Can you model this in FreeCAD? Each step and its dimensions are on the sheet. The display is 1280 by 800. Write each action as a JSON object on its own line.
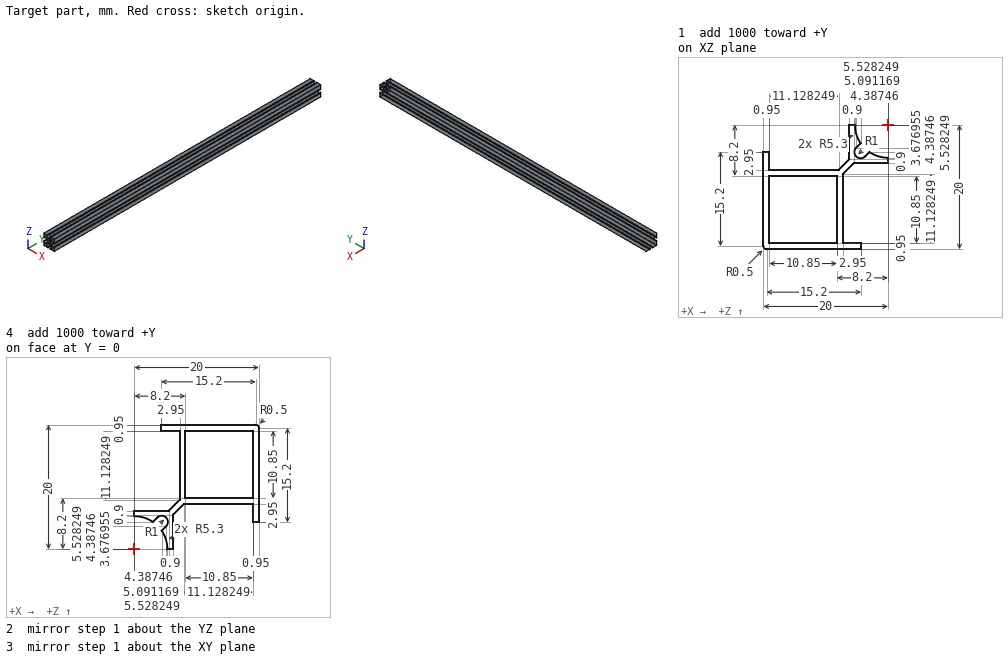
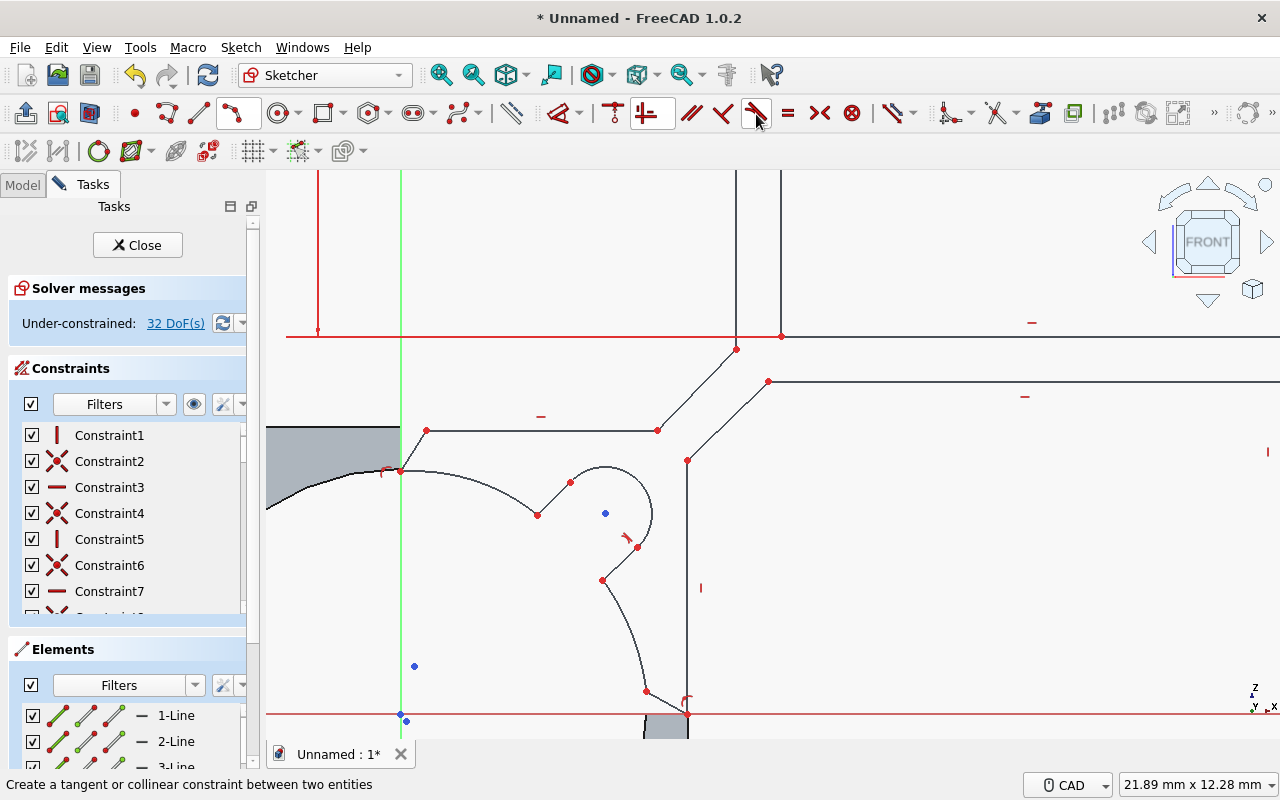
{"action": "left_click", "coordinate": [561, 492]}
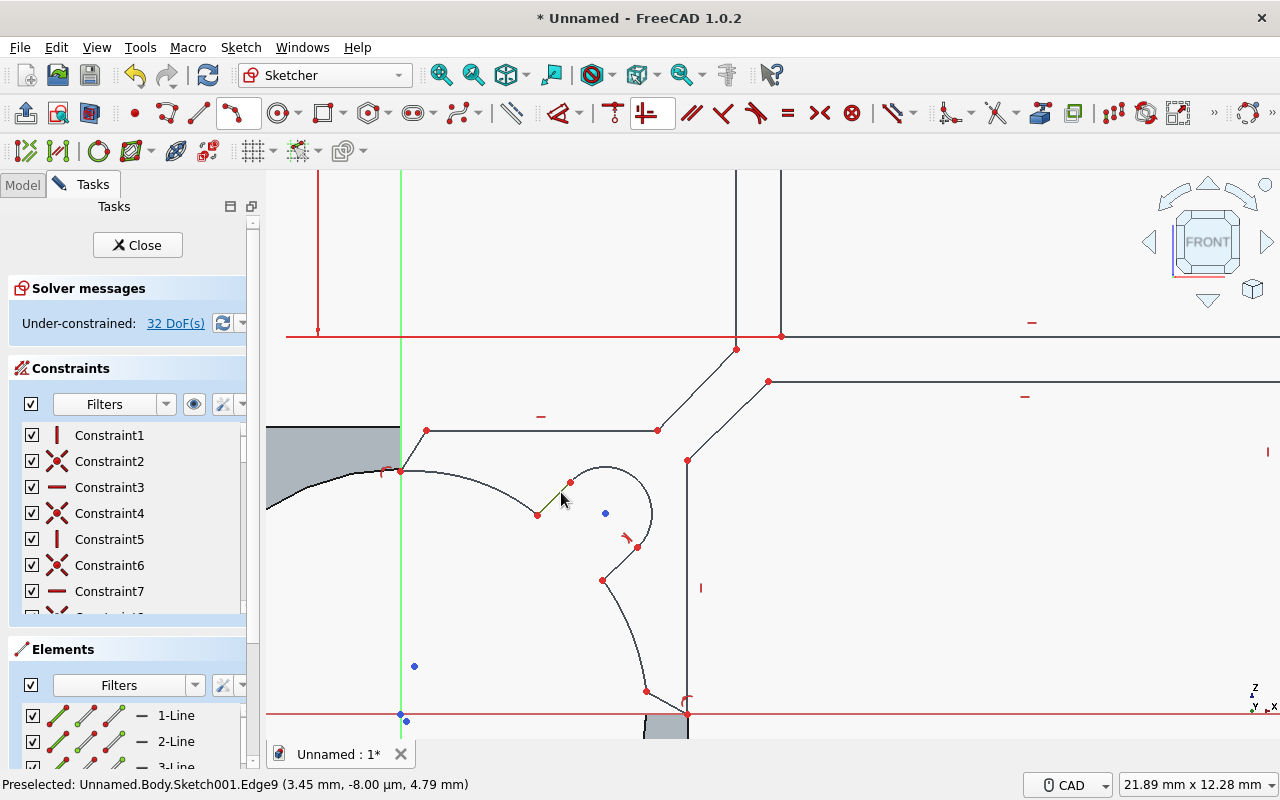
{"action": "left_click", "coordinate": [651, 507]}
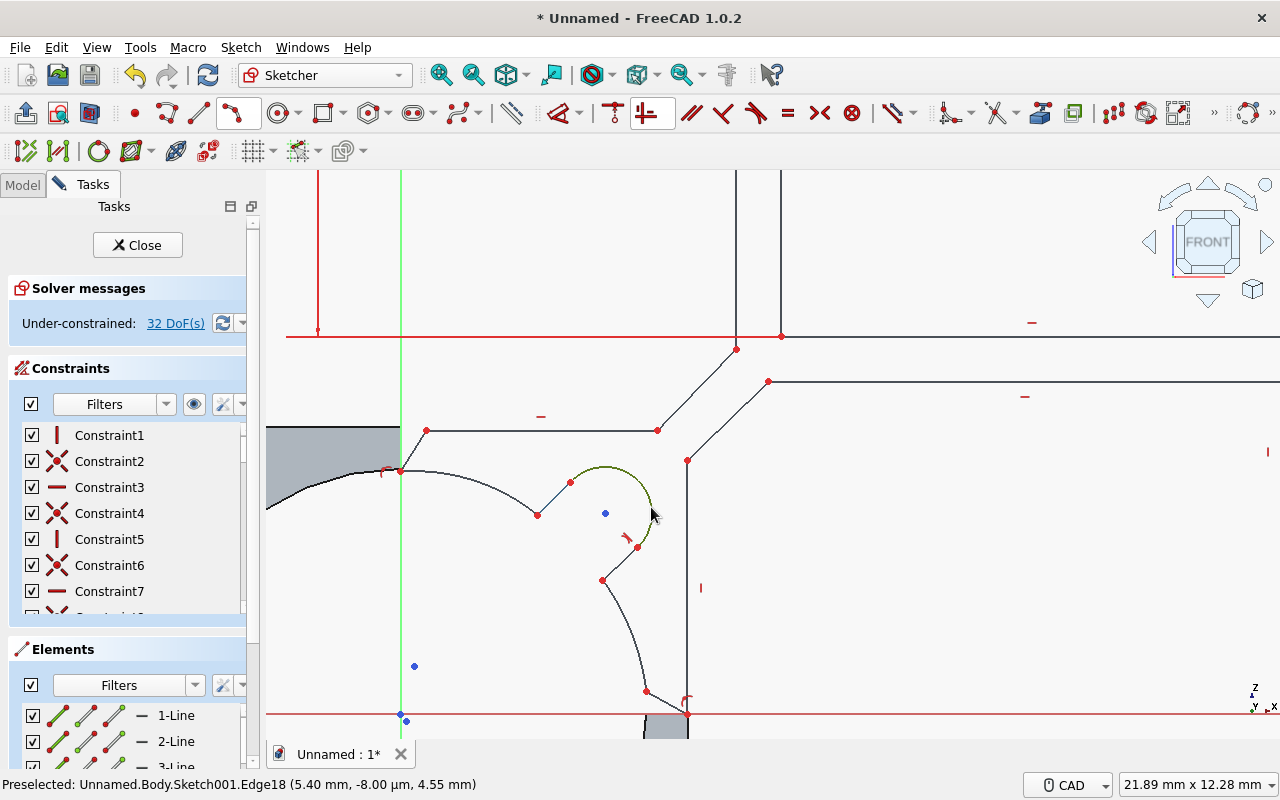
{"action": "left_click", "coordinate": [756, 114]}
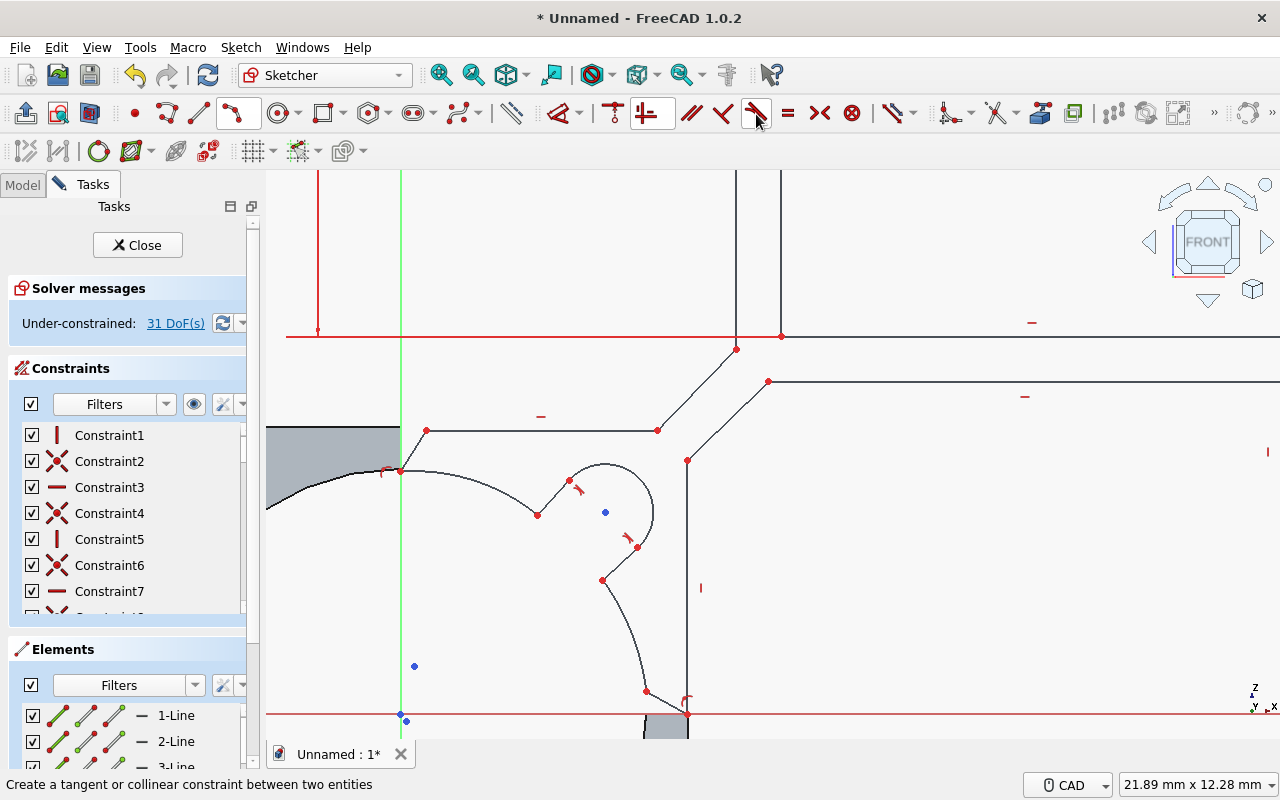
{"action": "scroll", "coordinate": [612, 573], "scroll_direction": "down", "scroll_amount": 5}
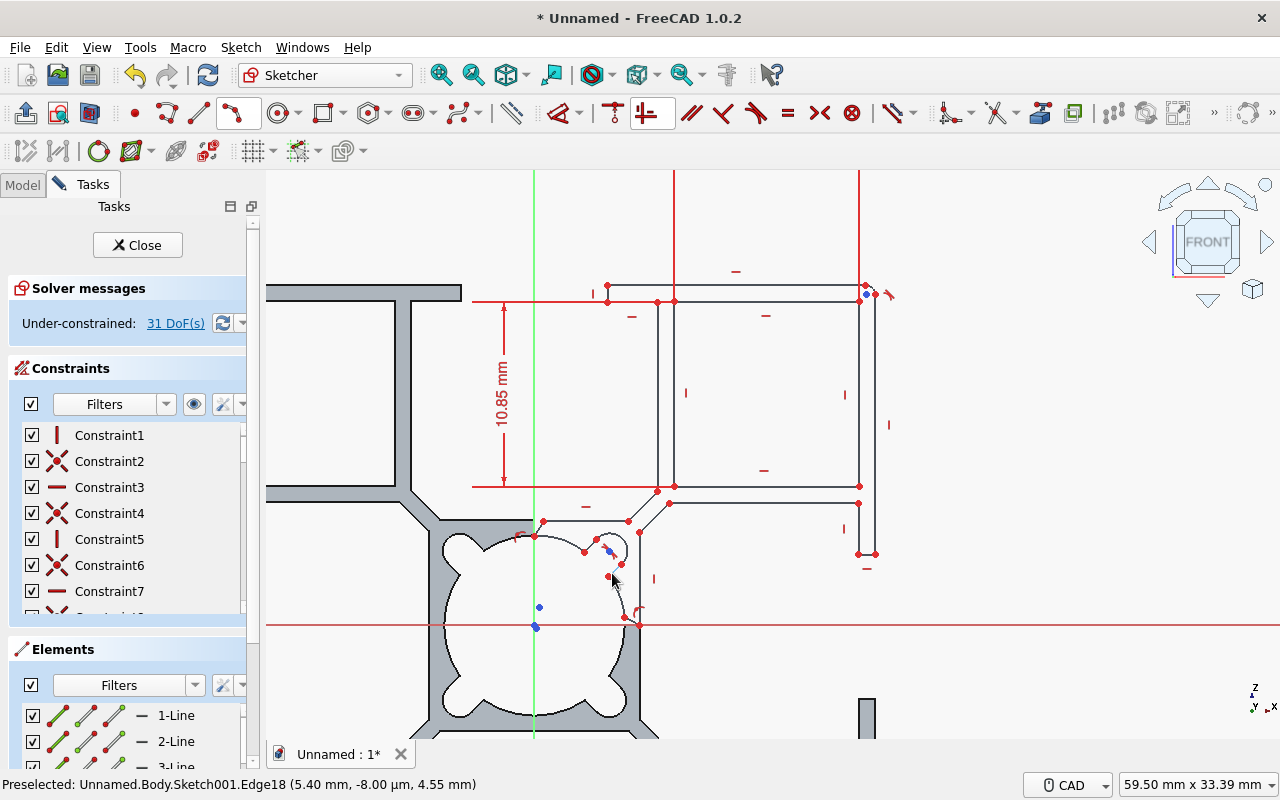
{"action": "left_click", "coordinate": [685, 285]}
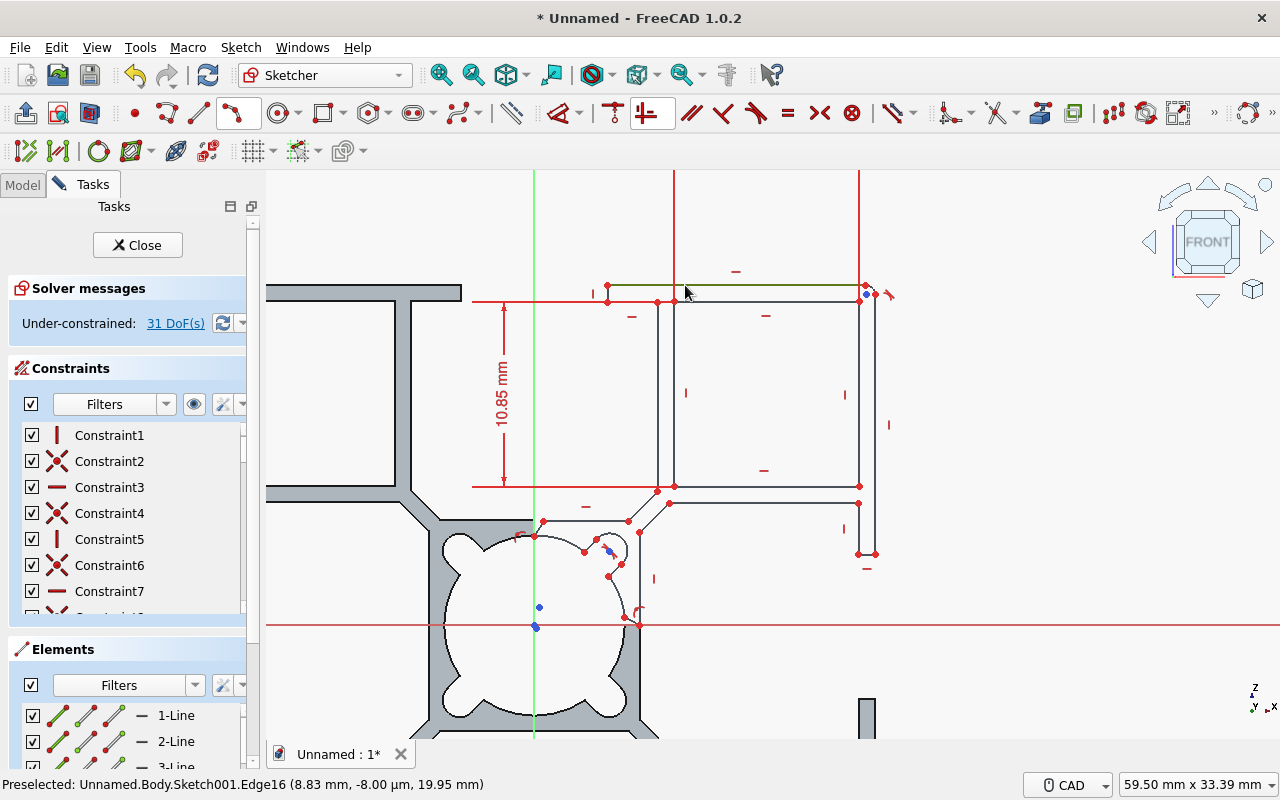
{"action": "scroll", "coordinate": [872, 288], "scroll_direction": "up", "scroll_amount": 4}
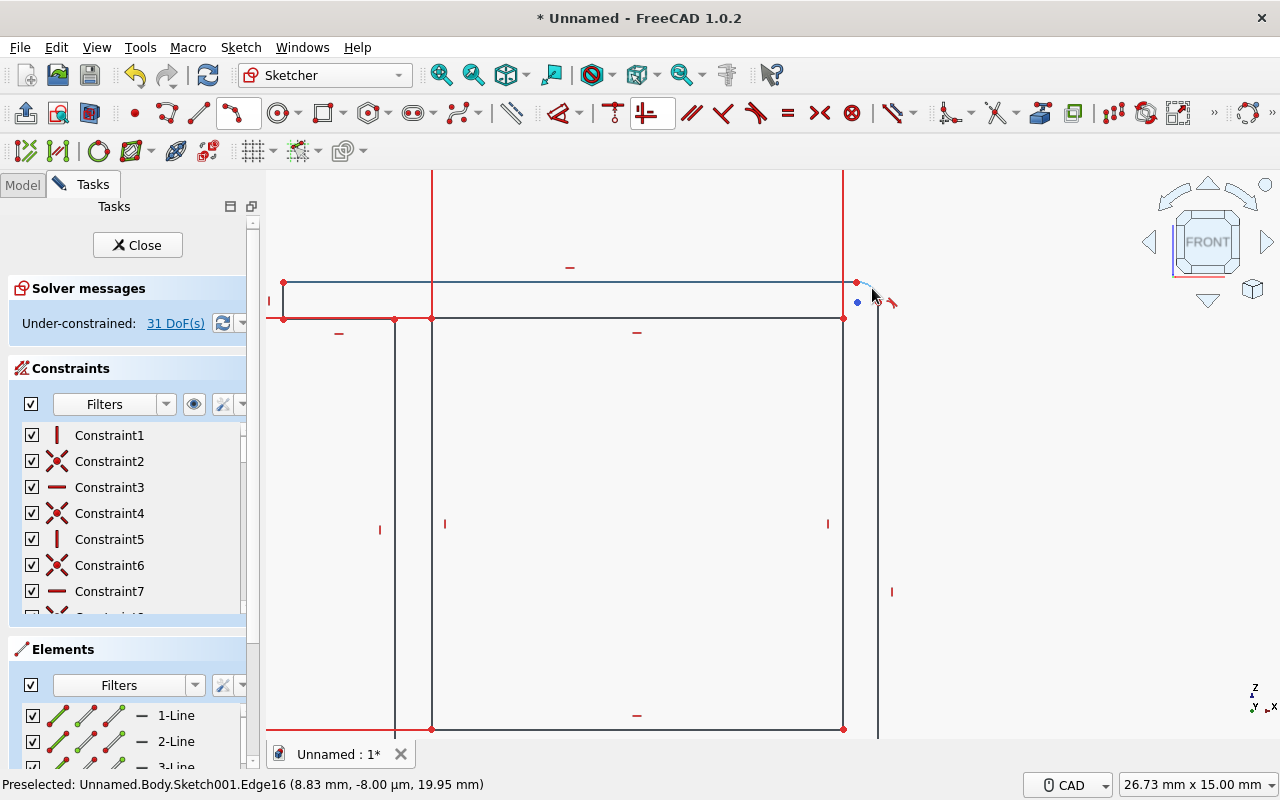
{"action": "left_click", "coordinate": [872, 288]}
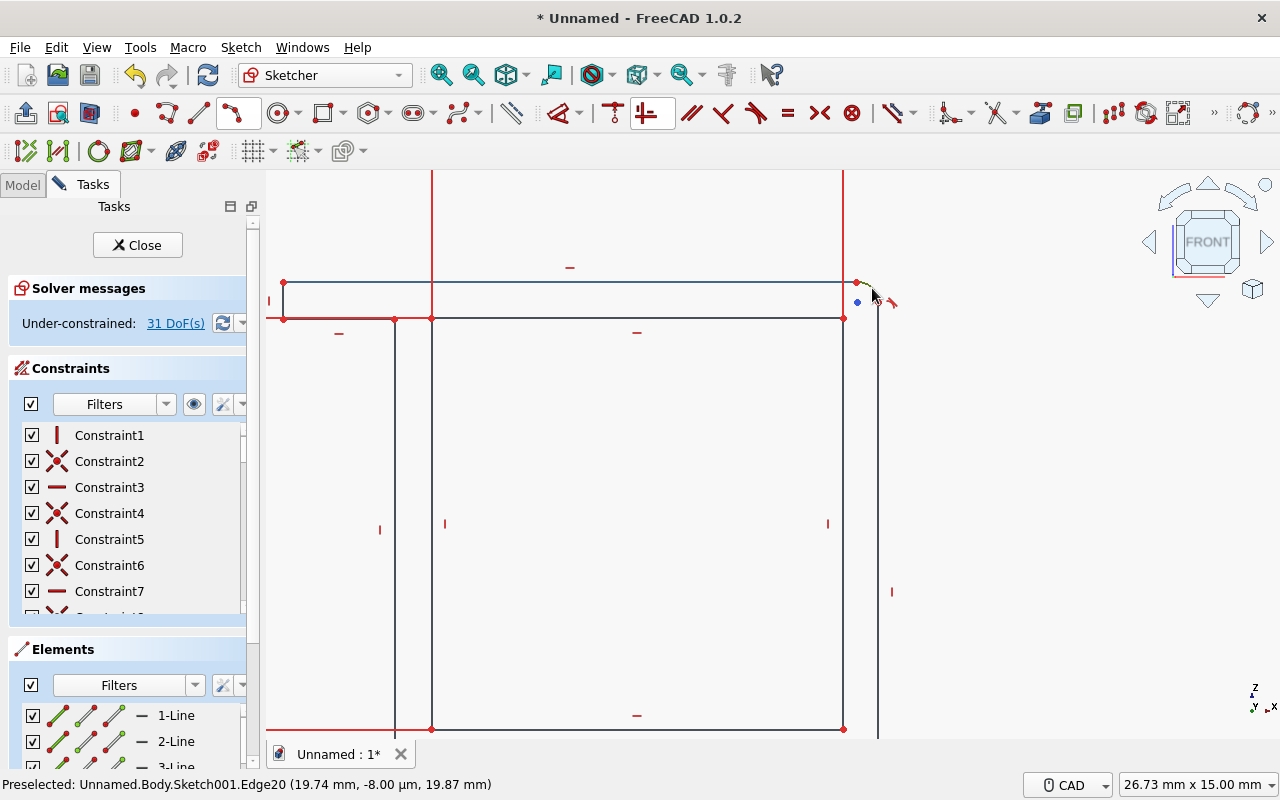
{"action": "left_click", "coordinate": [756, 114]}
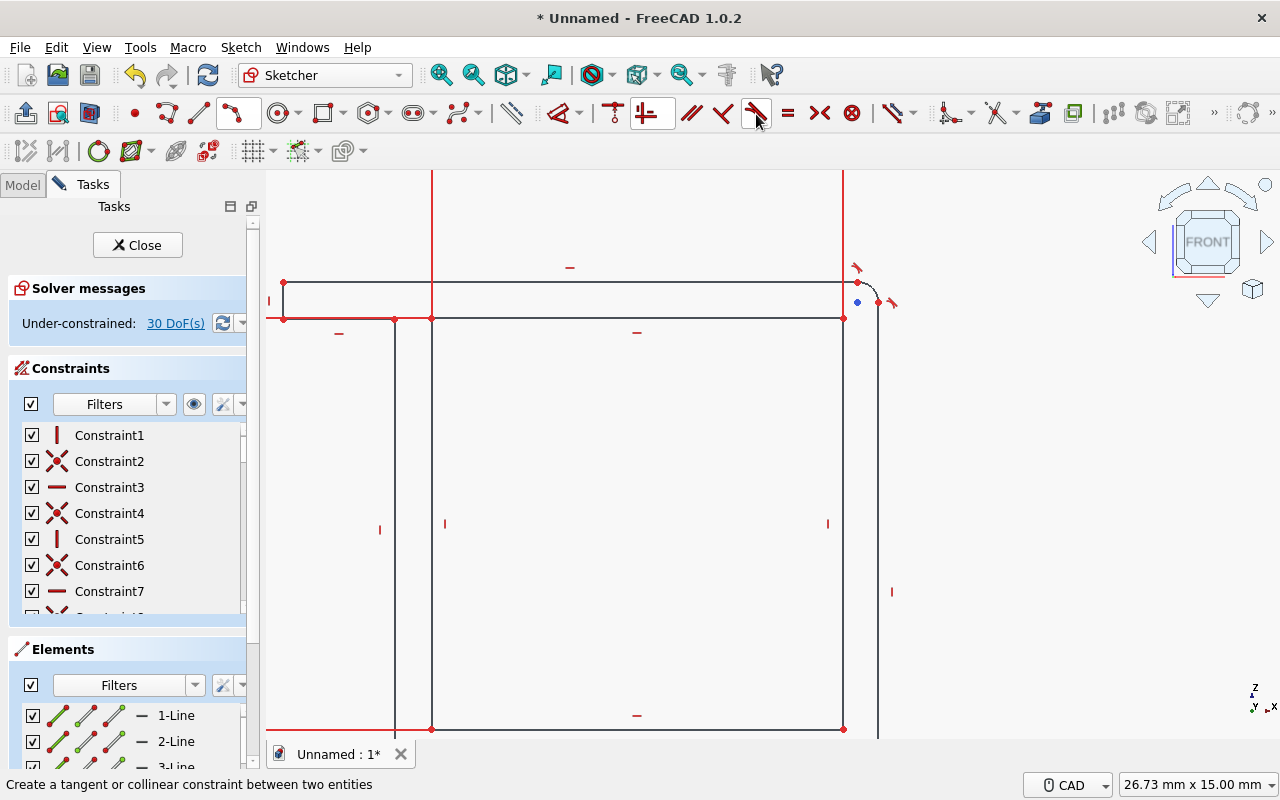
{"action": "scroll", "coordinate": [872, 287], "scroll_direction": "down", "scroll_amount": 4}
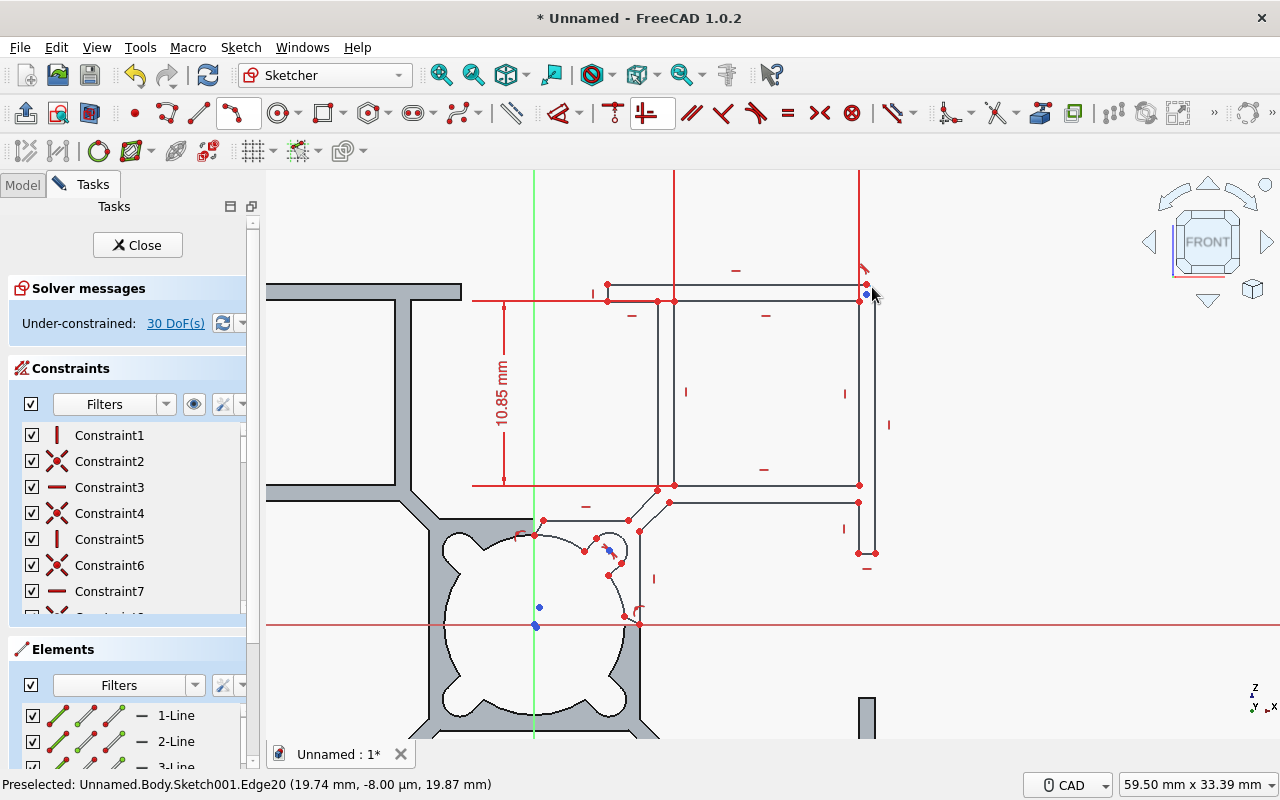
{"action": "scroll", "coordinate": [629, 619], "scroll_direction": "up", "scroll_amount": 5}